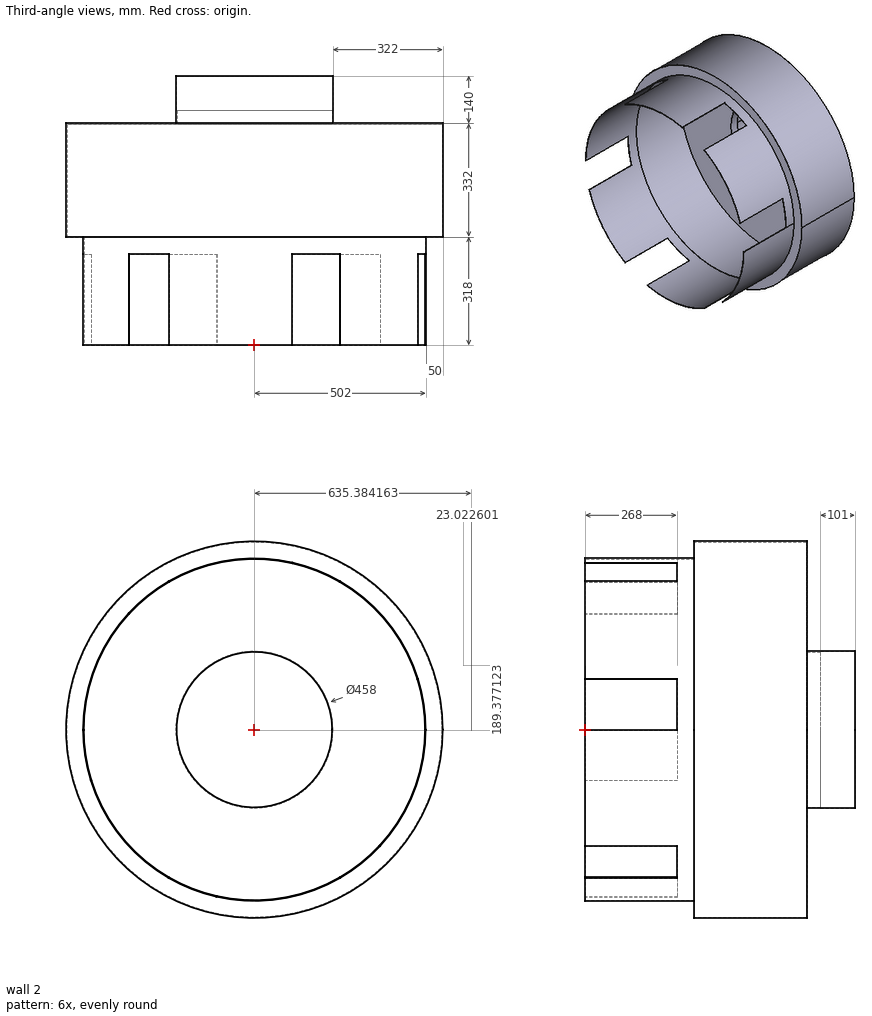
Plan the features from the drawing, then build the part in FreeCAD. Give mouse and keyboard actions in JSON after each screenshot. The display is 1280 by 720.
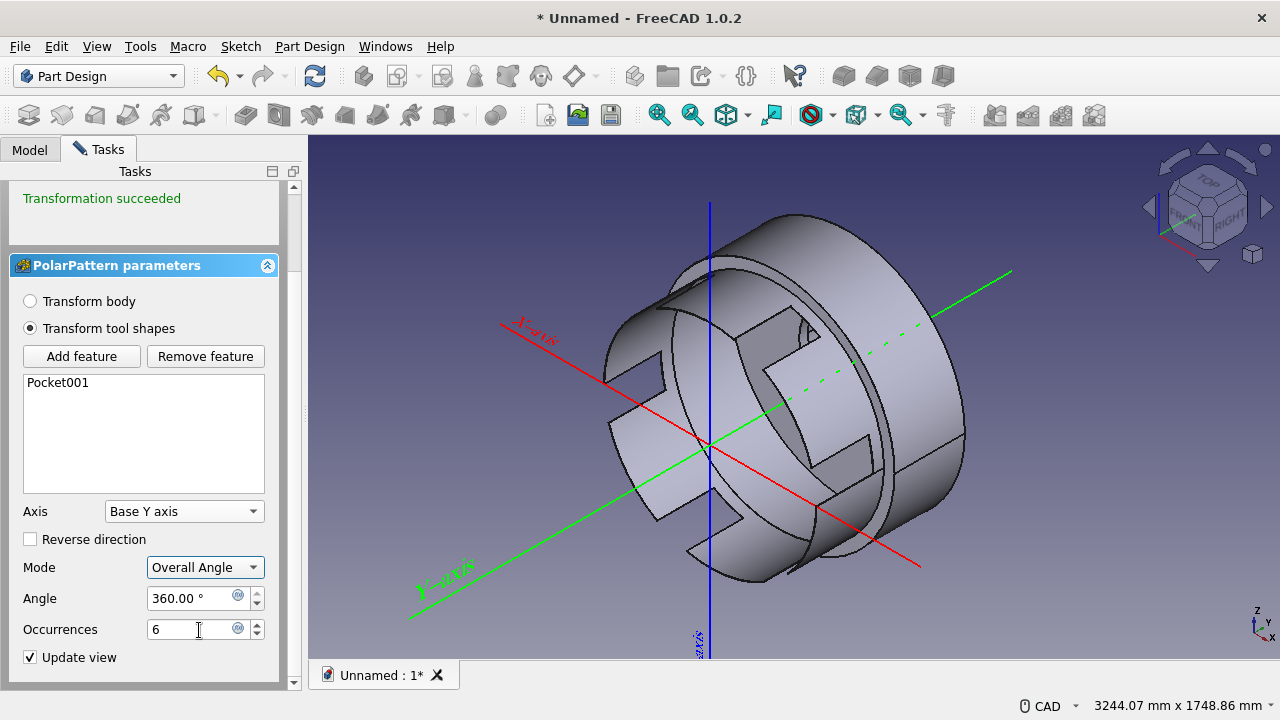
{"action": "scroll", "coordinate": [294, 436], "scroll_direction": "up", "scroll_amount": 3}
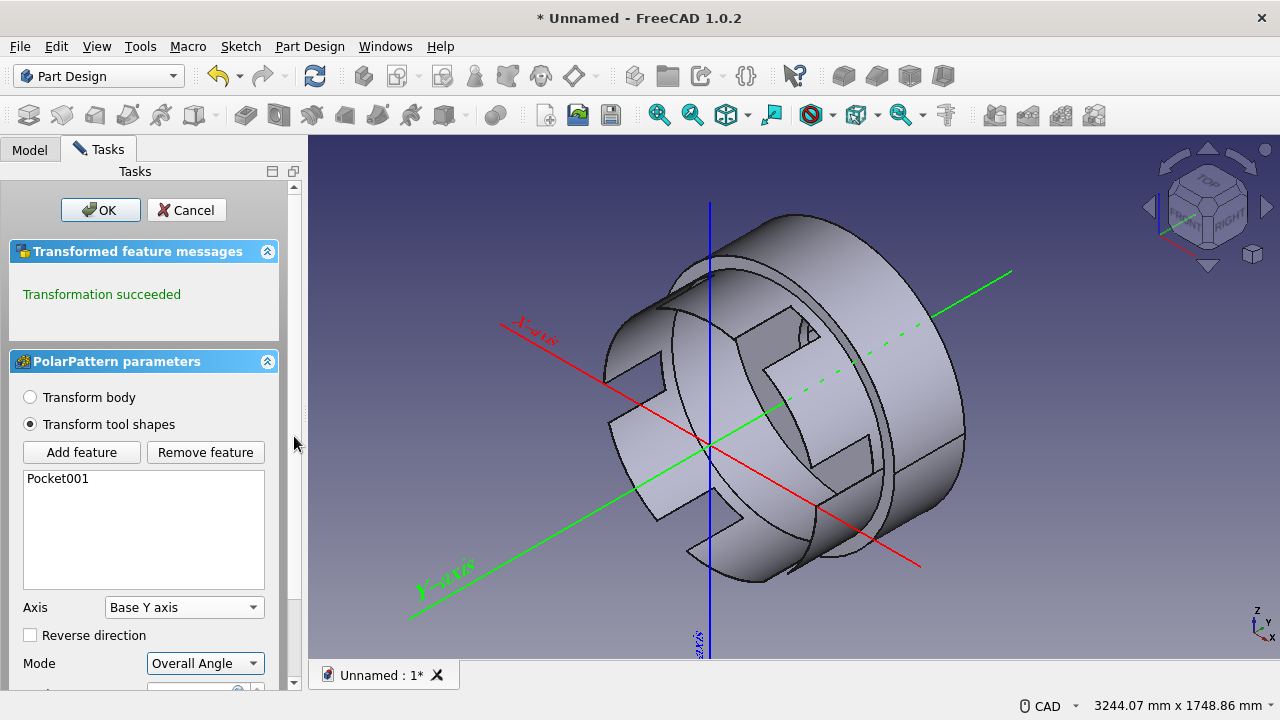
{"action": "left_click", "coordinate": [101, 210]}